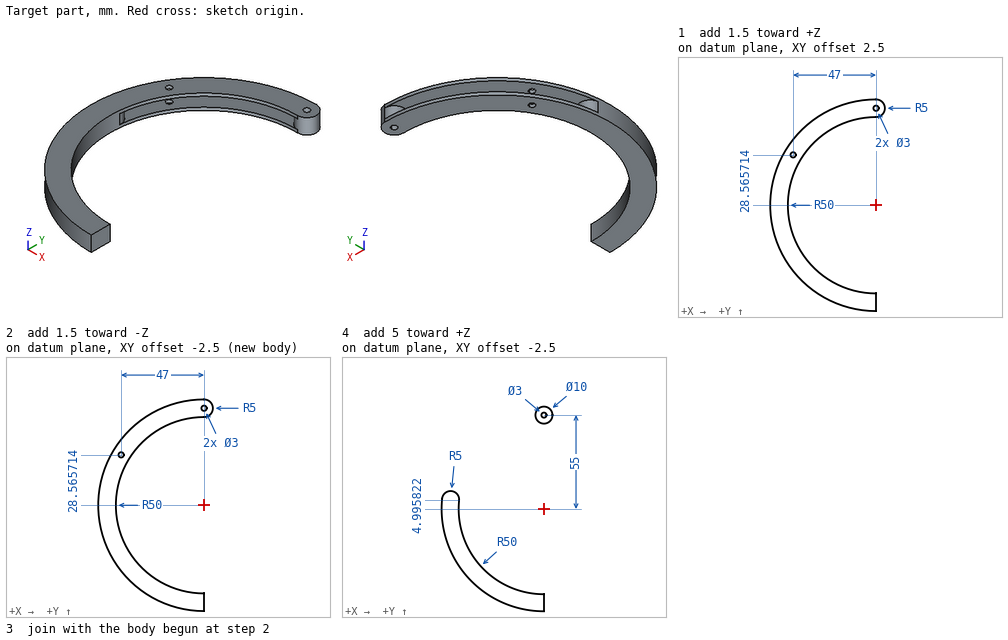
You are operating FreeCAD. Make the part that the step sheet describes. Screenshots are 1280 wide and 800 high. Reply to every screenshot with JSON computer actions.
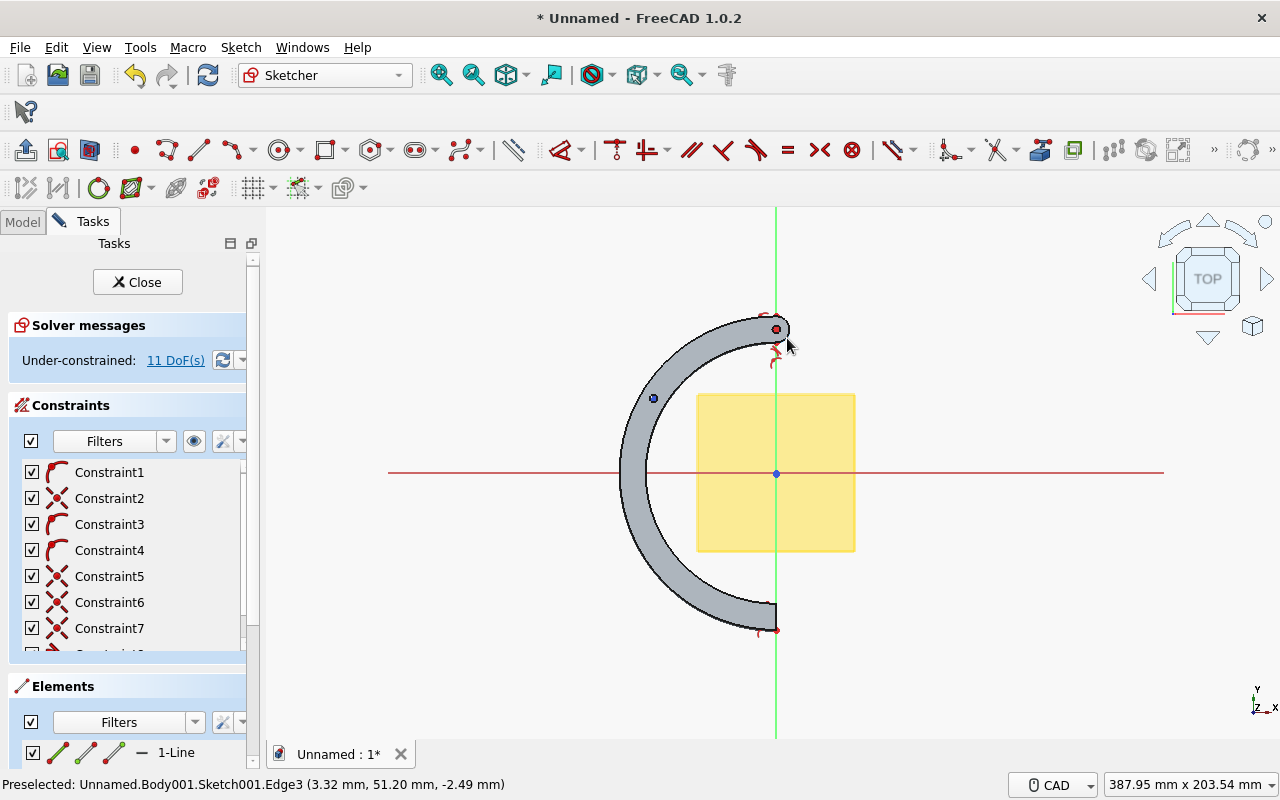
{"action": "scroll", "coordinate": [770, 613], "scroll_direction": "up", "scroll_amount": 4}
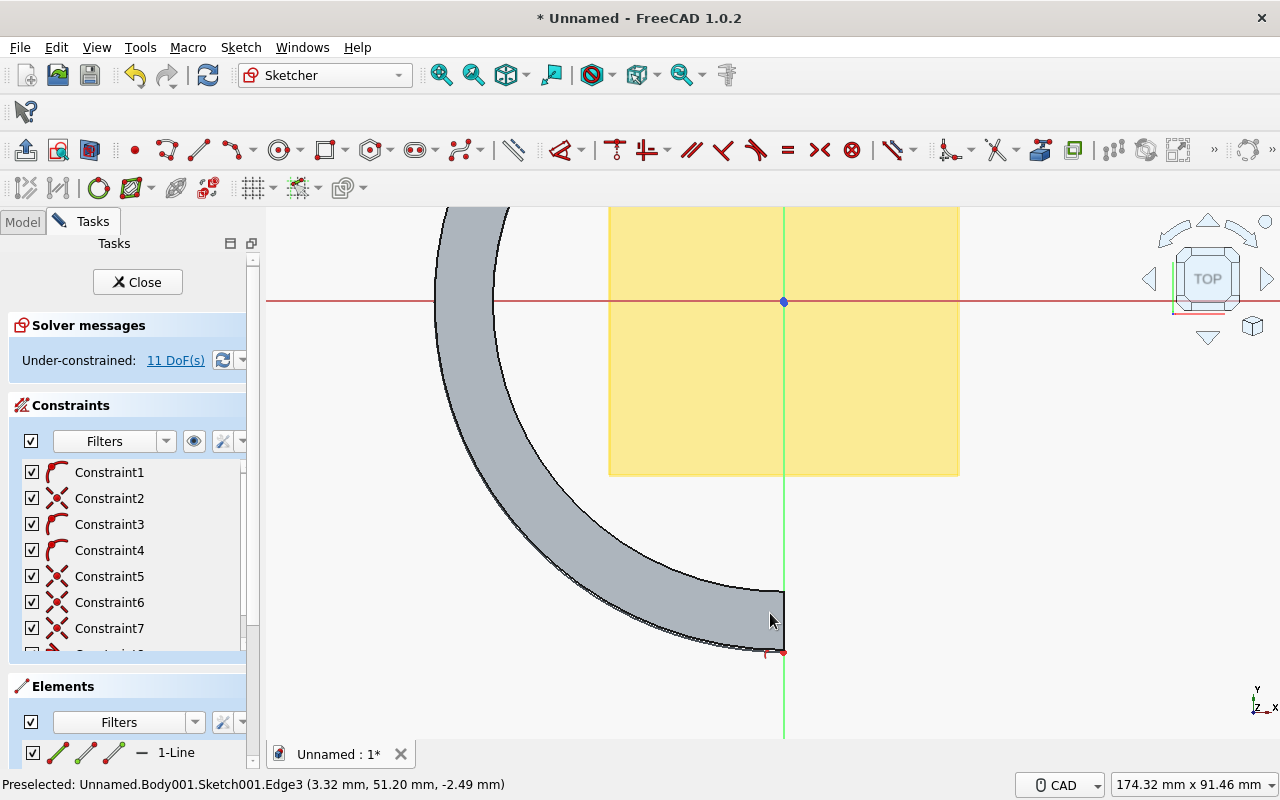
{"action": "left_click", "coordinate": [769, 612]}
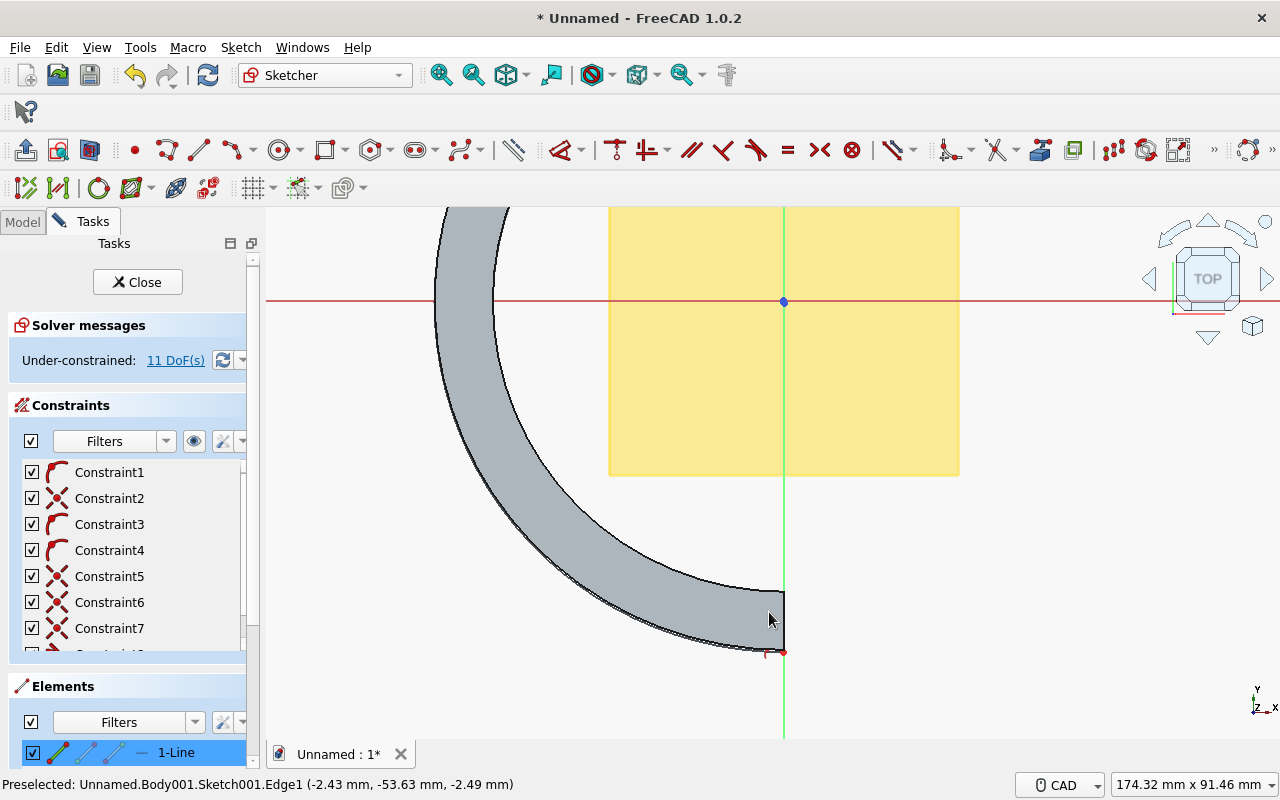
{"action": "key", "text": "v"}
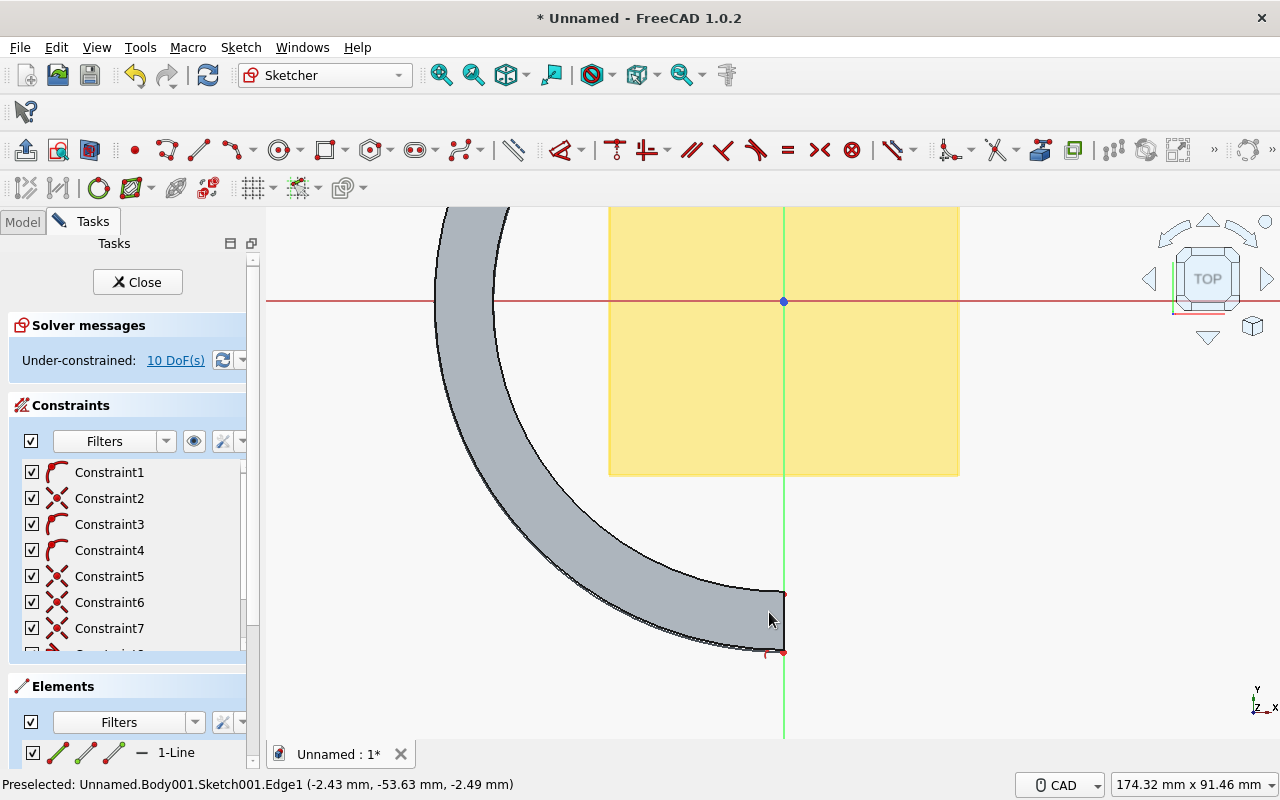
{"action": "left_click", "coordinate": [549, 474]}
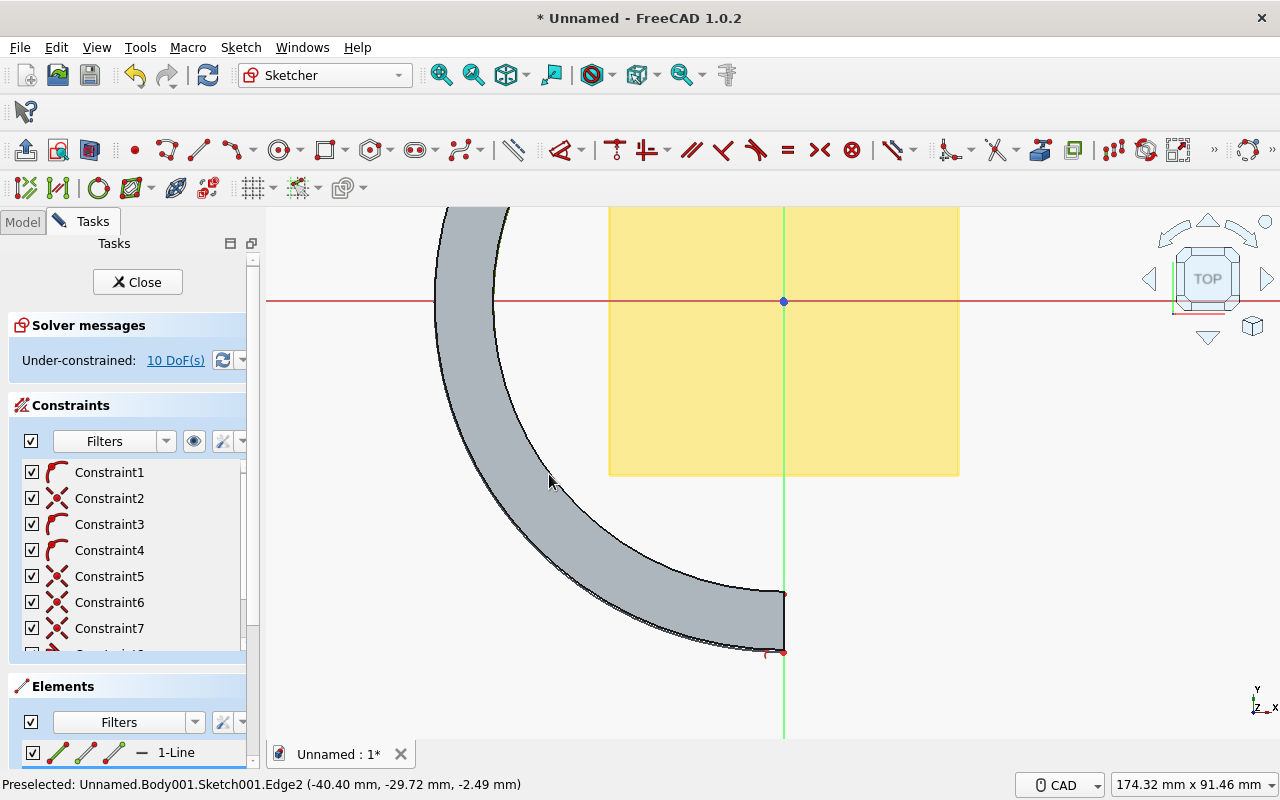
{"action": "left_click", "coordinate": [501, 508]}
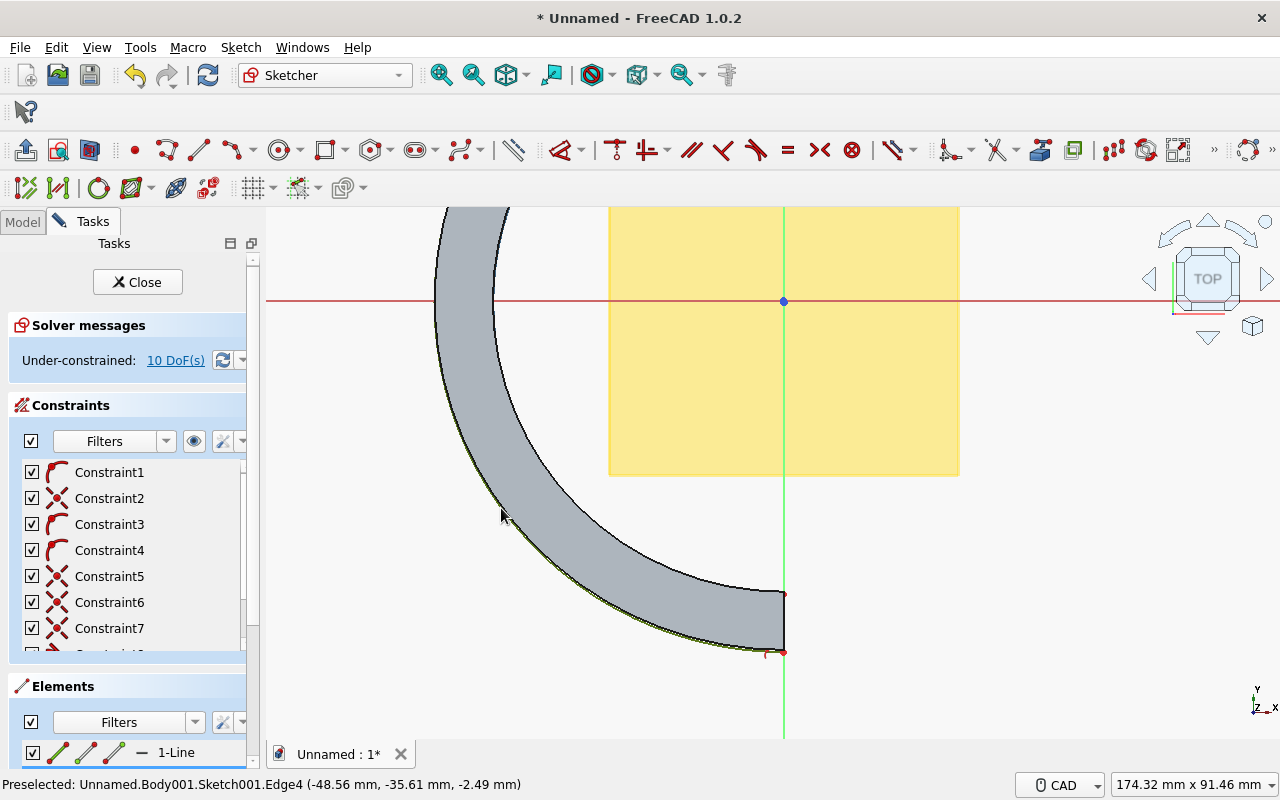
{"action": "left_click", "coordinate": [616, 150]}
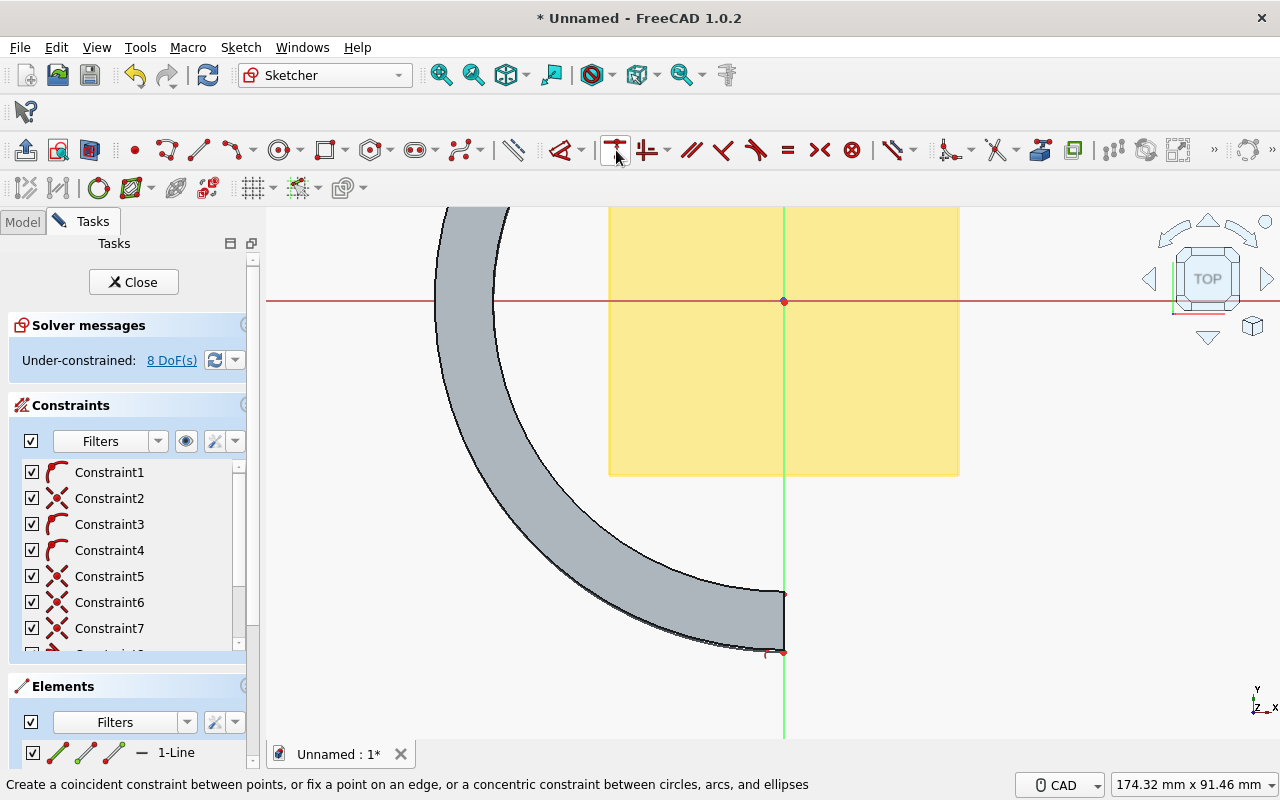
{"action": "scroll", "coordinate": [784, 302], "scroll_direction": "up", "scroll_amount": 9}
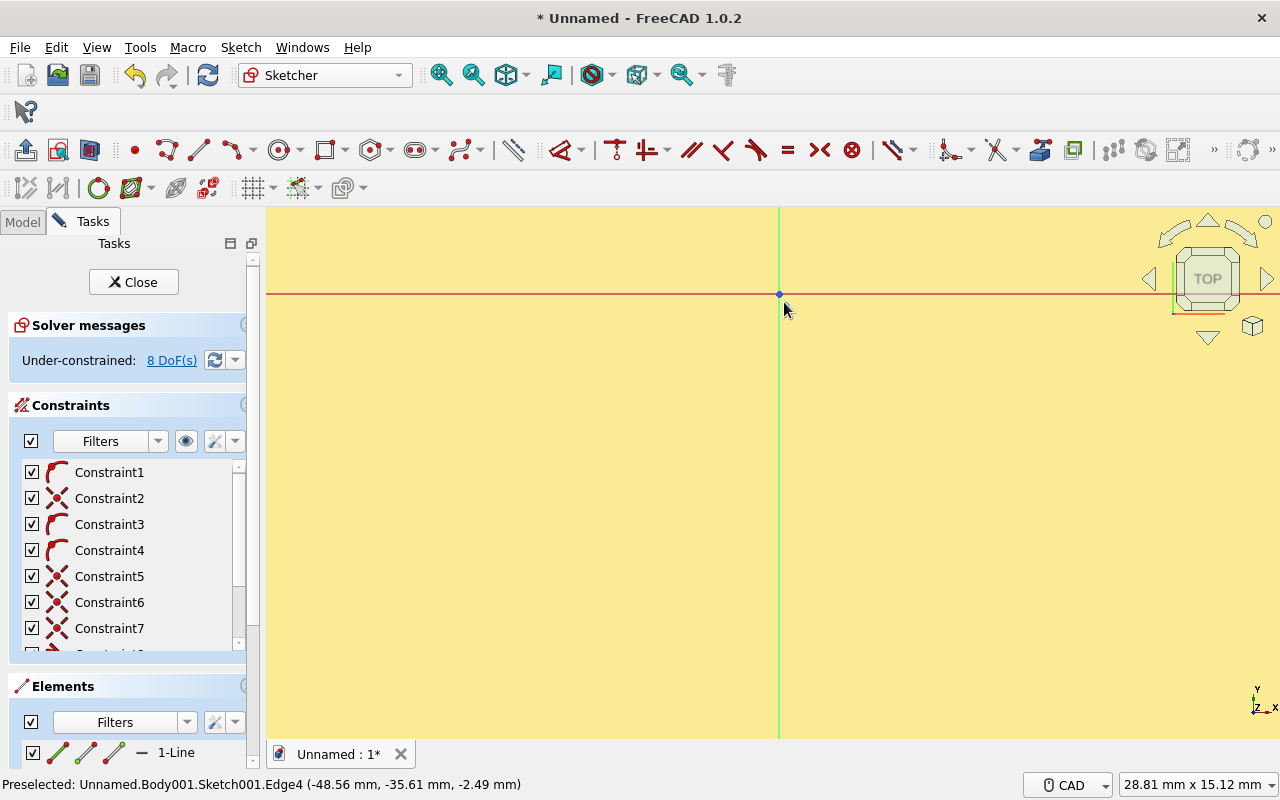
{"action": "left_click_drag", "start_coordinate": [769, 284], "coordinate": [796, 315]}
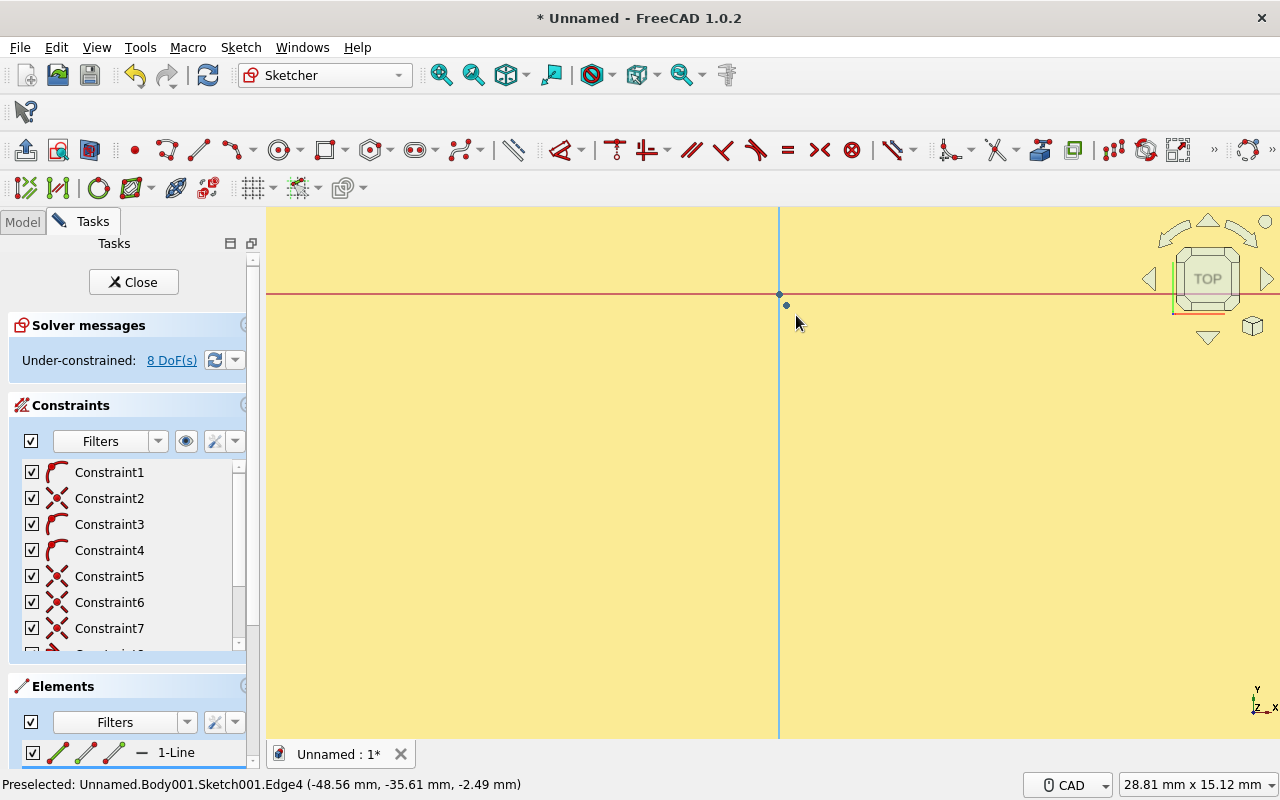
{"action": "left_click", "coordinate": [616, 150]}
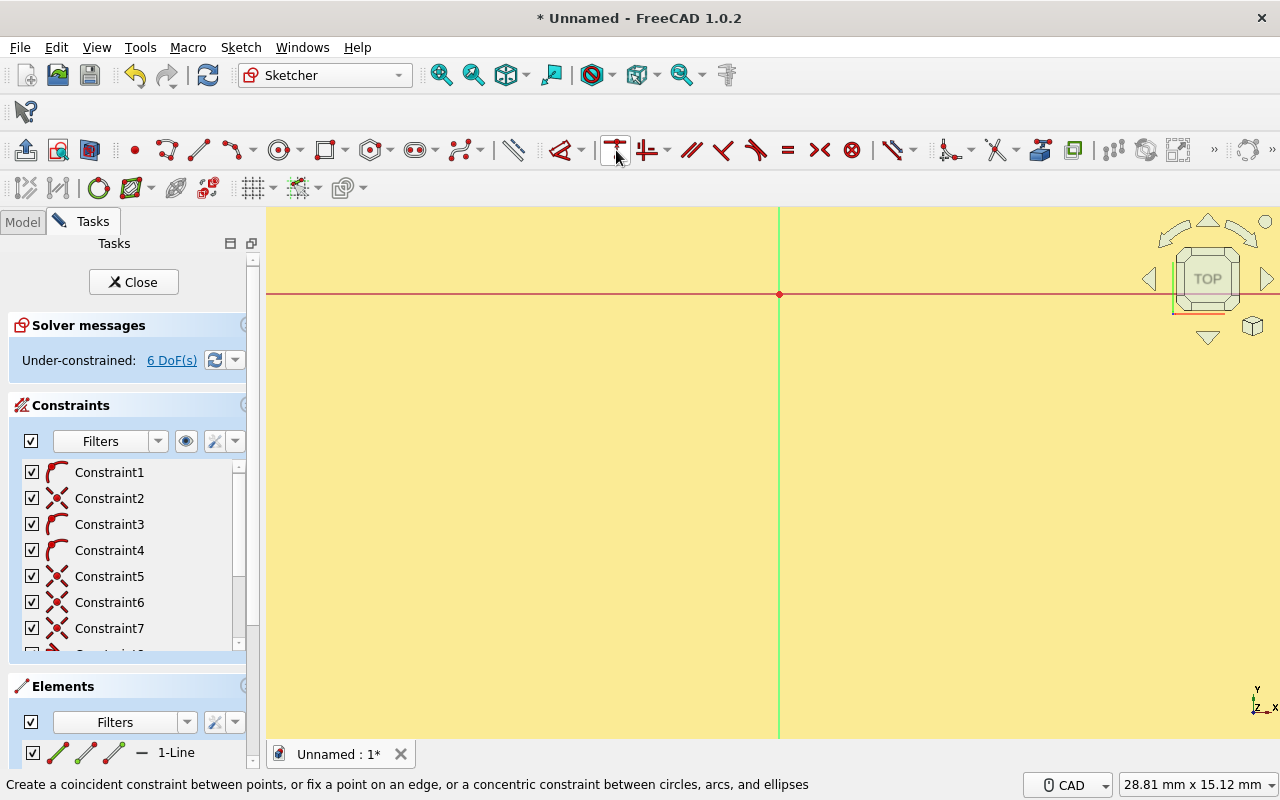
{"action": "scroll", "coordinate": [776, 487], "scroll_direction": "down", "scroll_amount": 13}